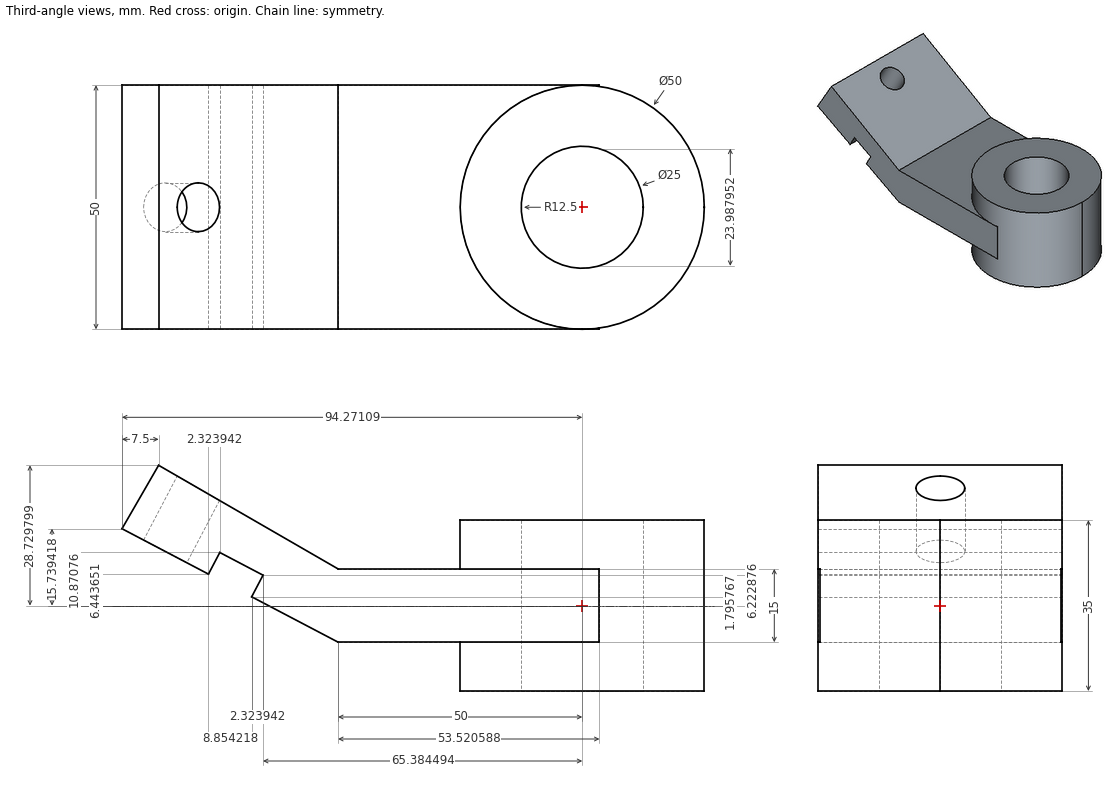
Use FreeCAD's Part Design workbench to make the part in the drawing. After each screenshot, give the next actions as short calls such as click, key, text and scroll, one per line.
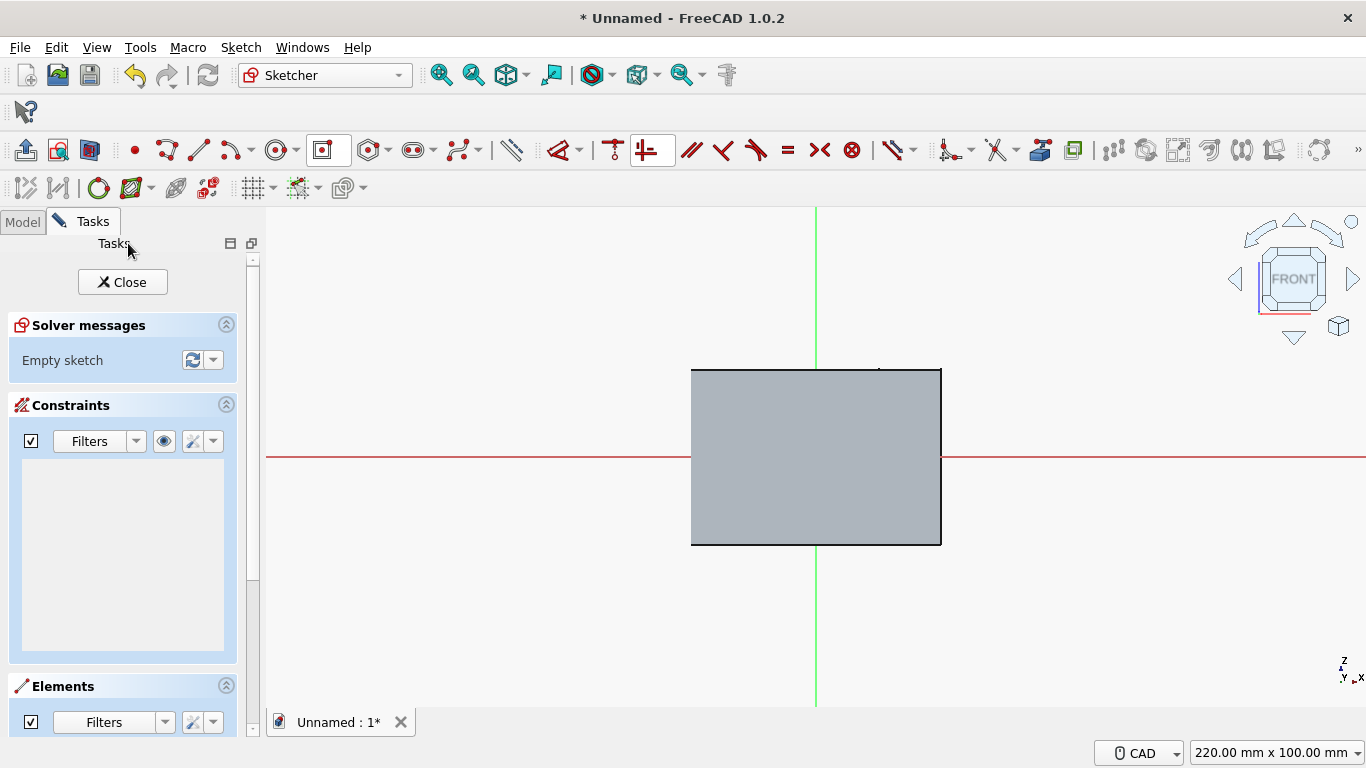
click(90, 150)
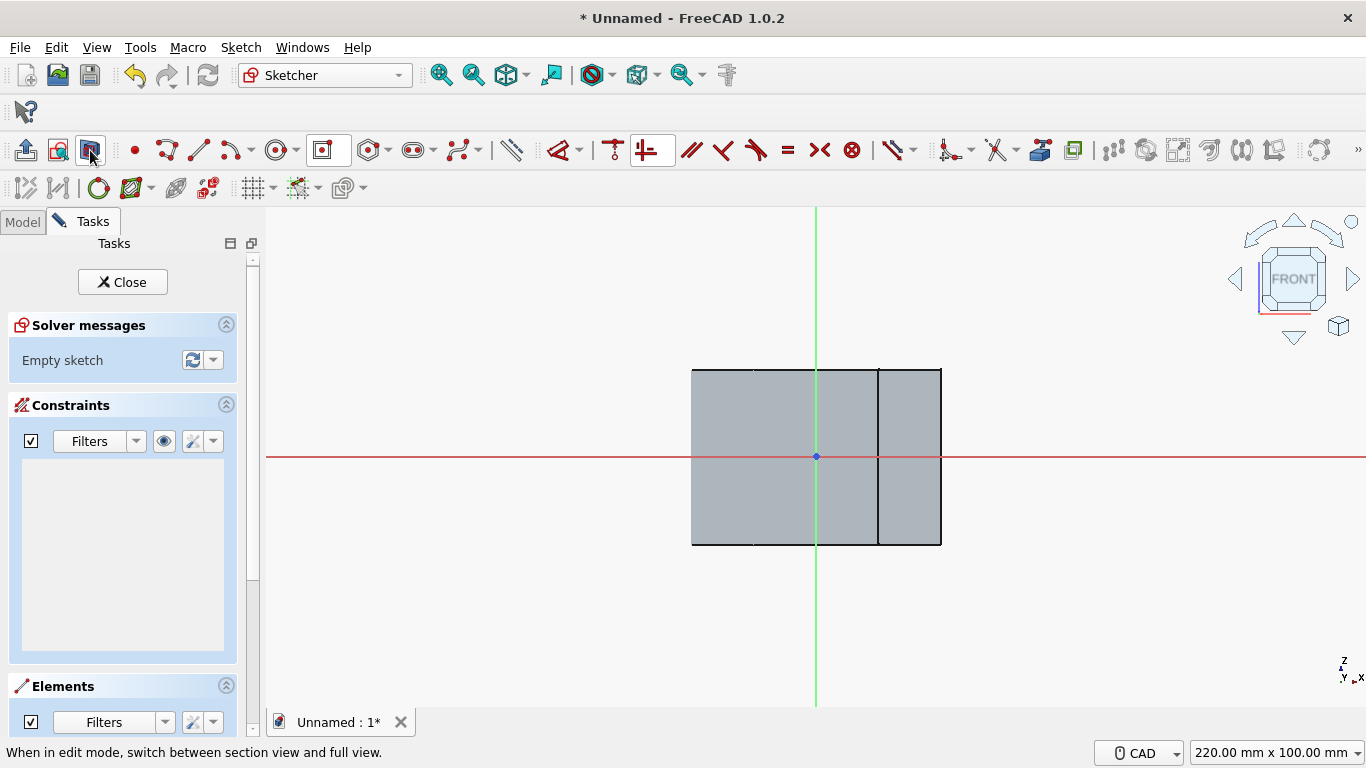
click(168, 150)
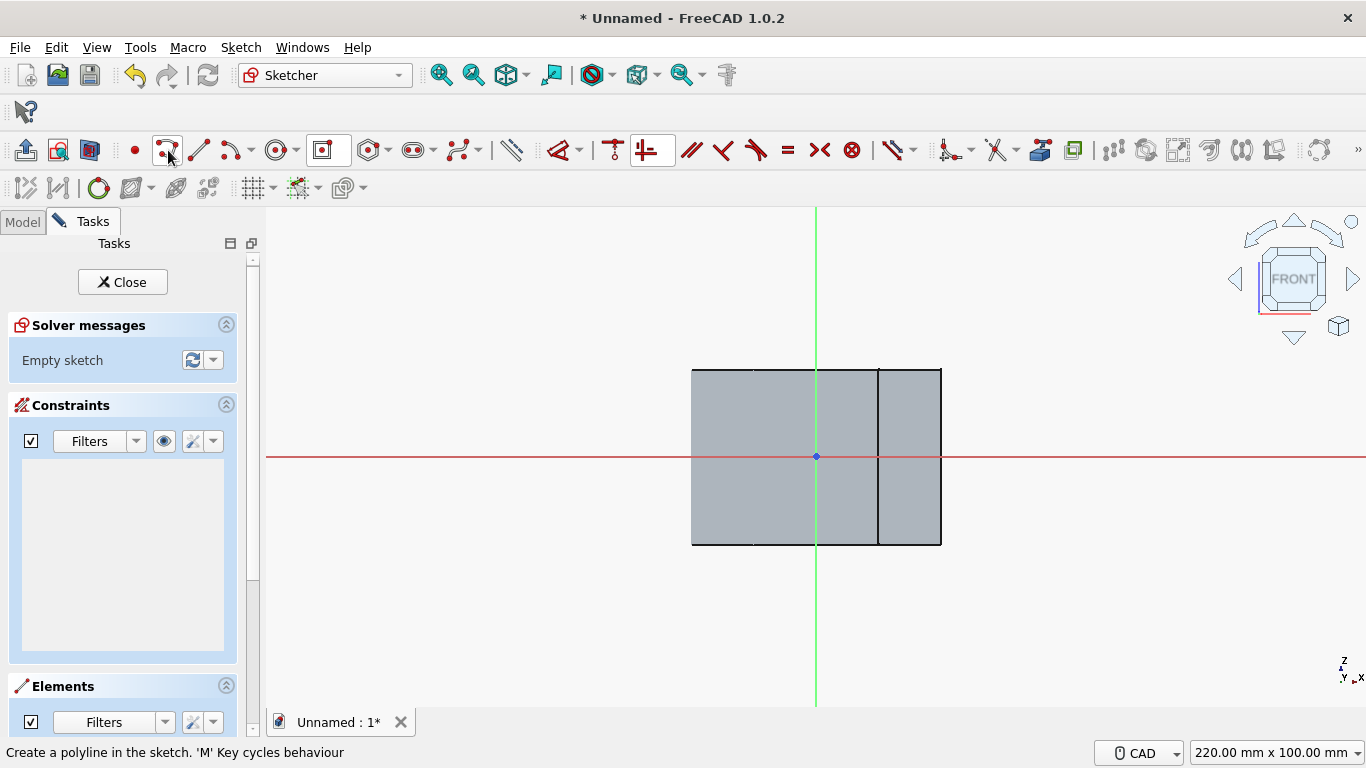
click(834, 494)
click(566, 494)
click(345, 378)
click(382, 313)
click(566, 420)
click(834, 420)
click(834, 495)
key(Escape)
key(Escape)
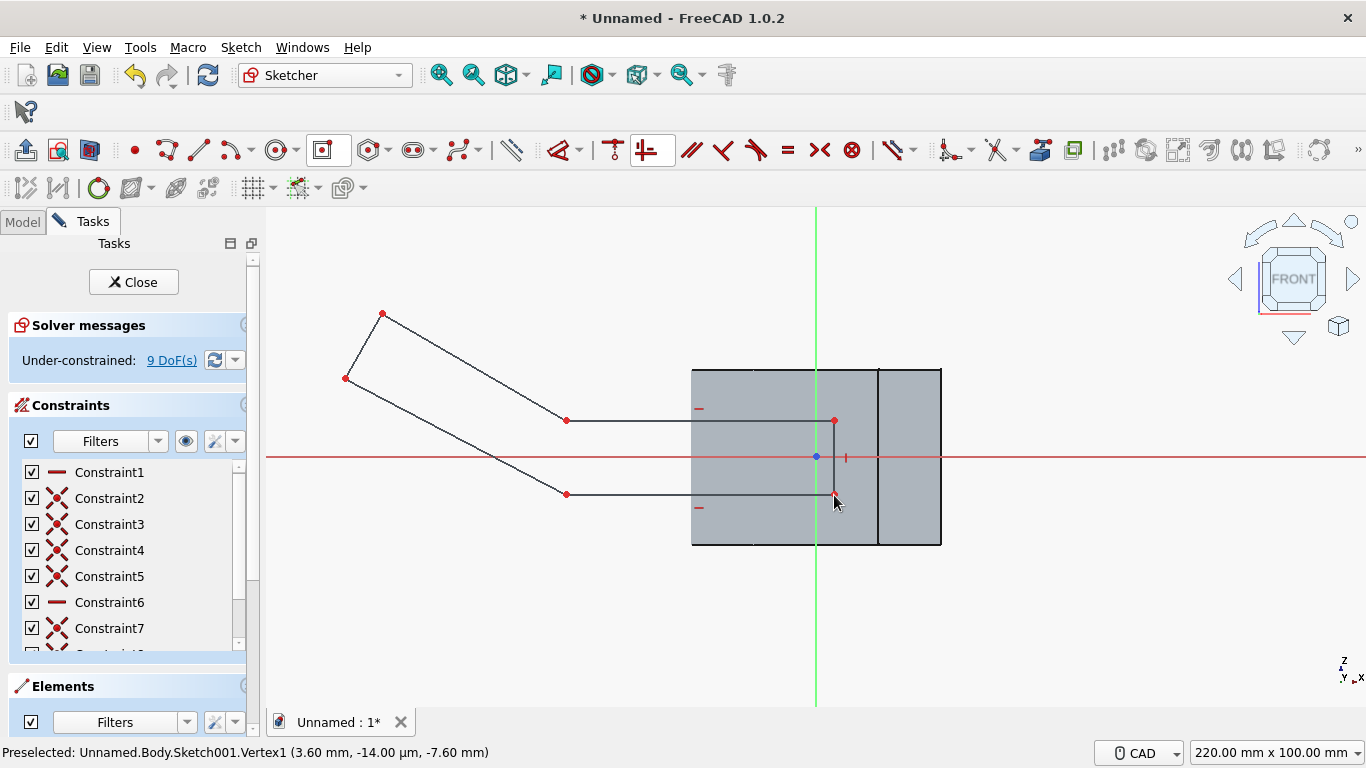
click(566, 495)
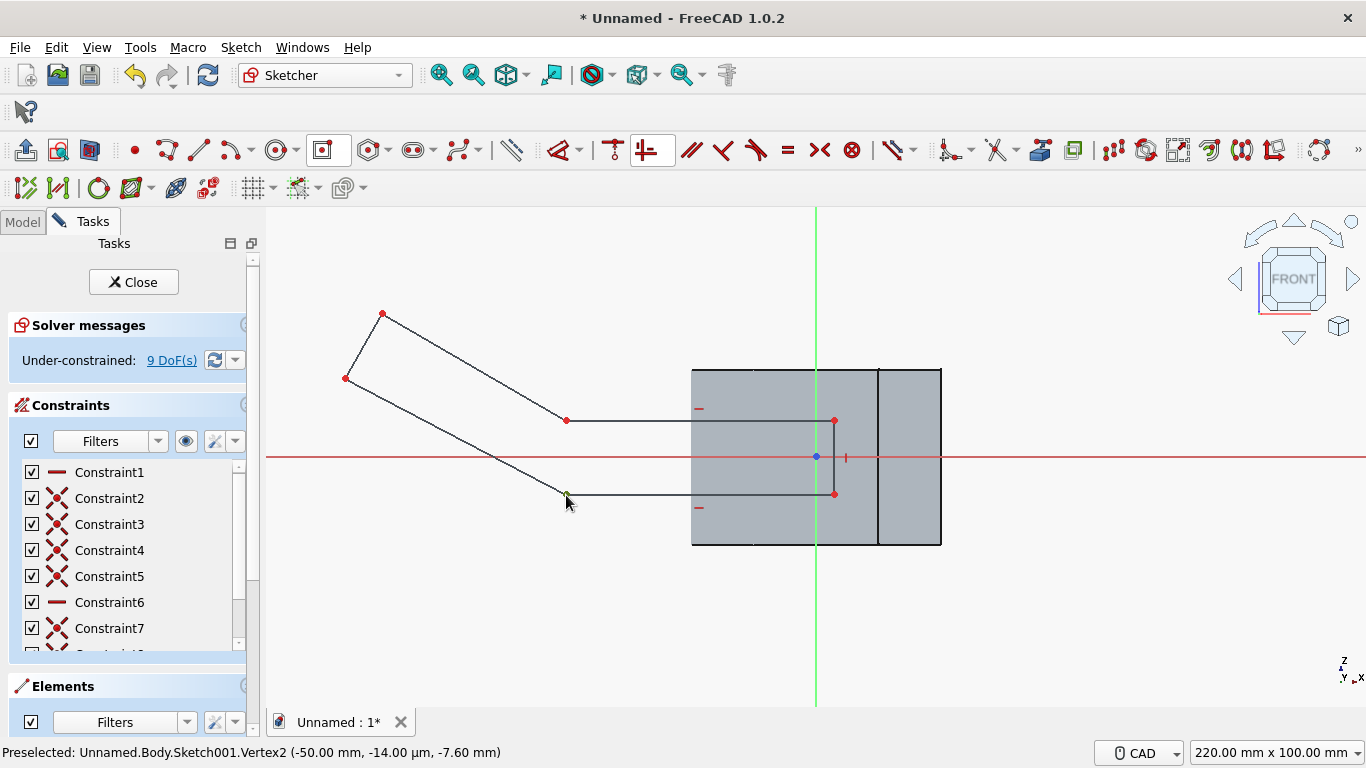
click(566, 421)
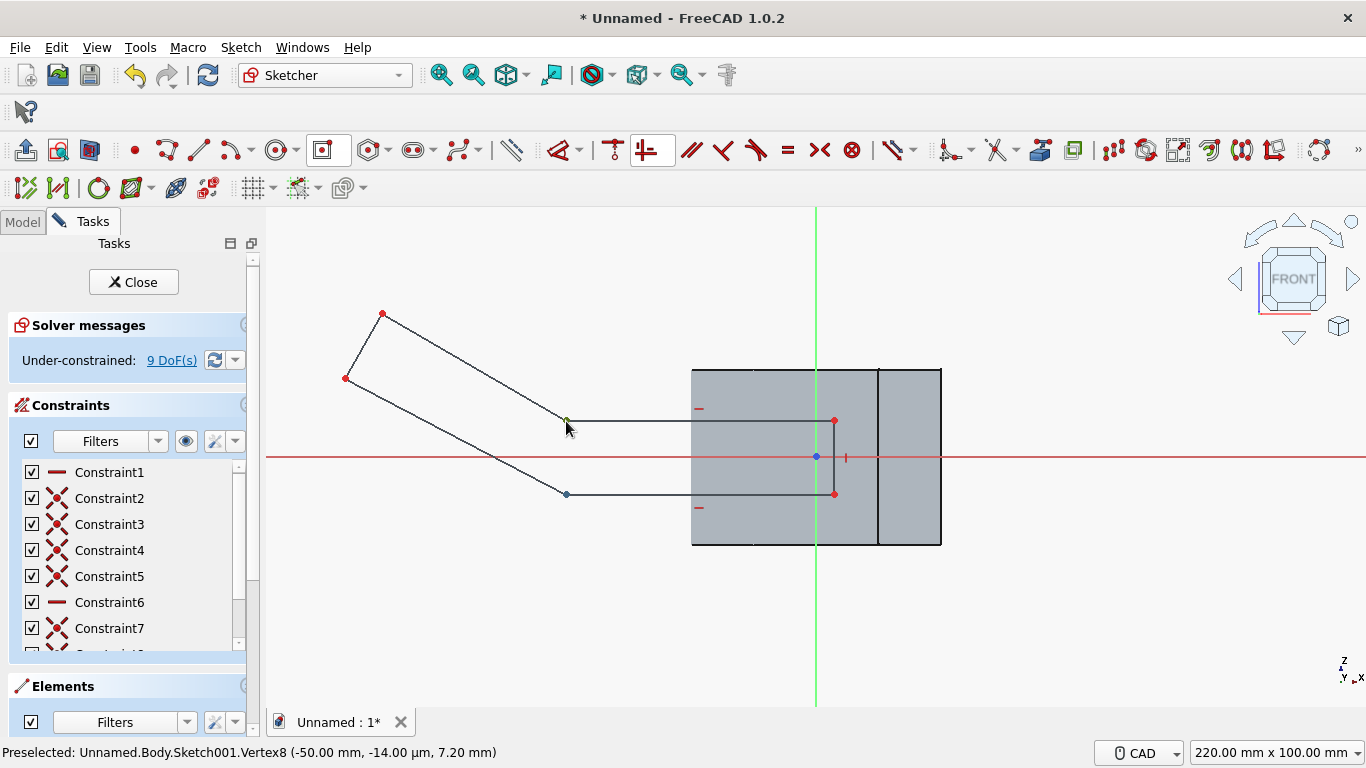
click(359, 457)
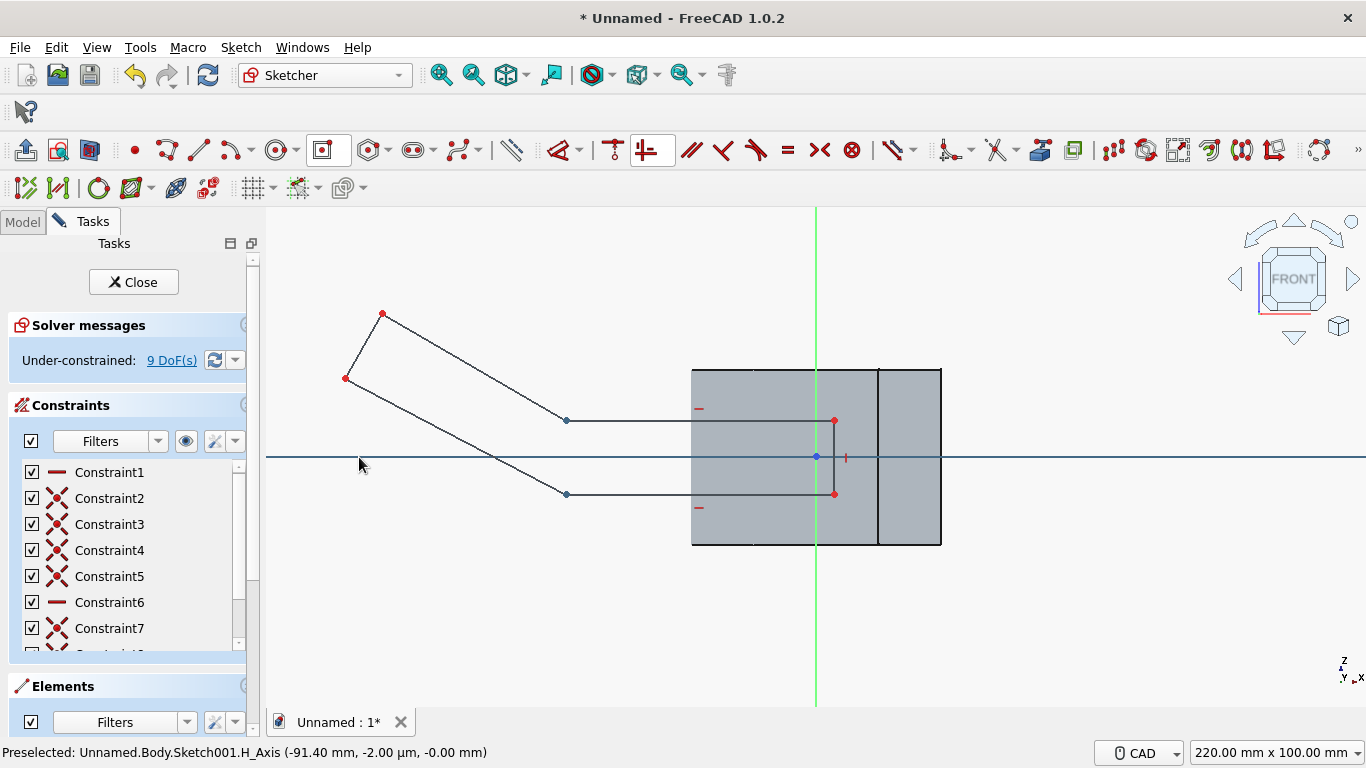
click(820, 150)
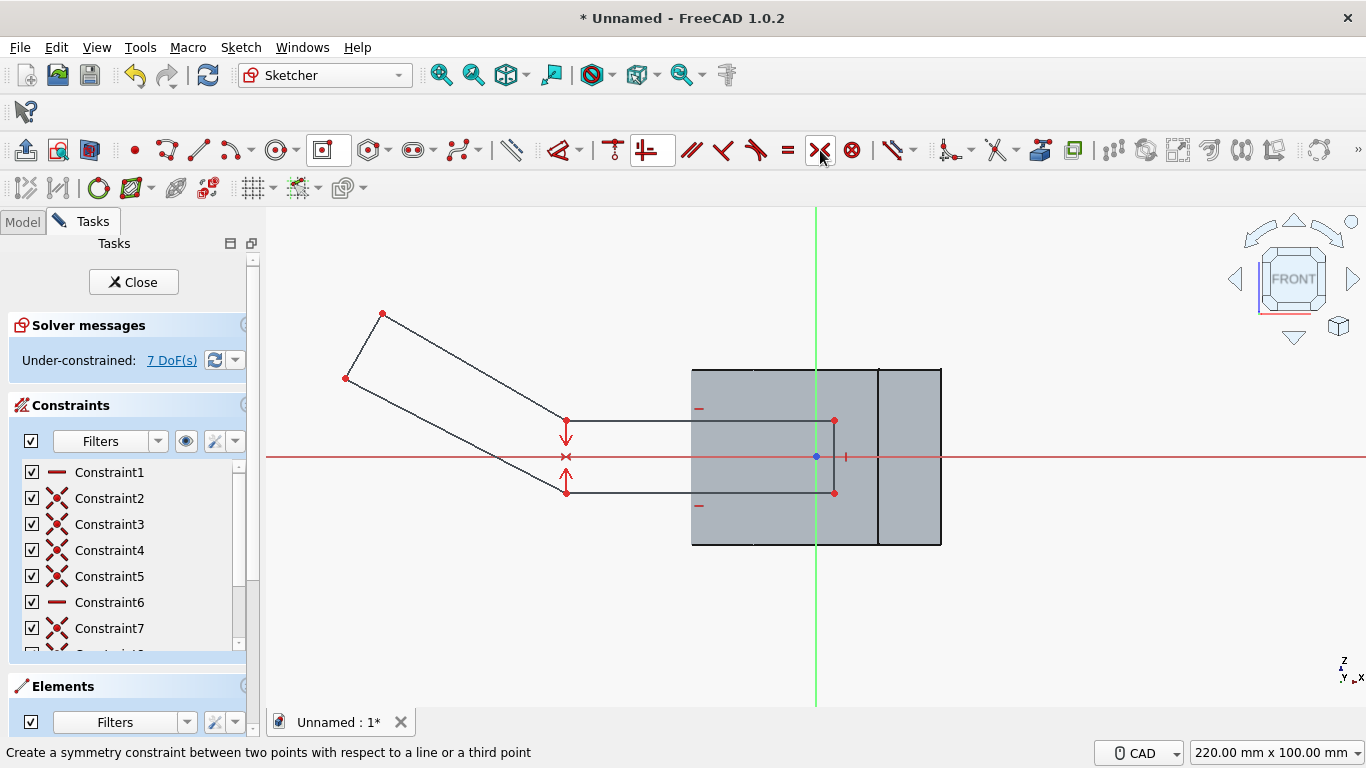
click(558, 150)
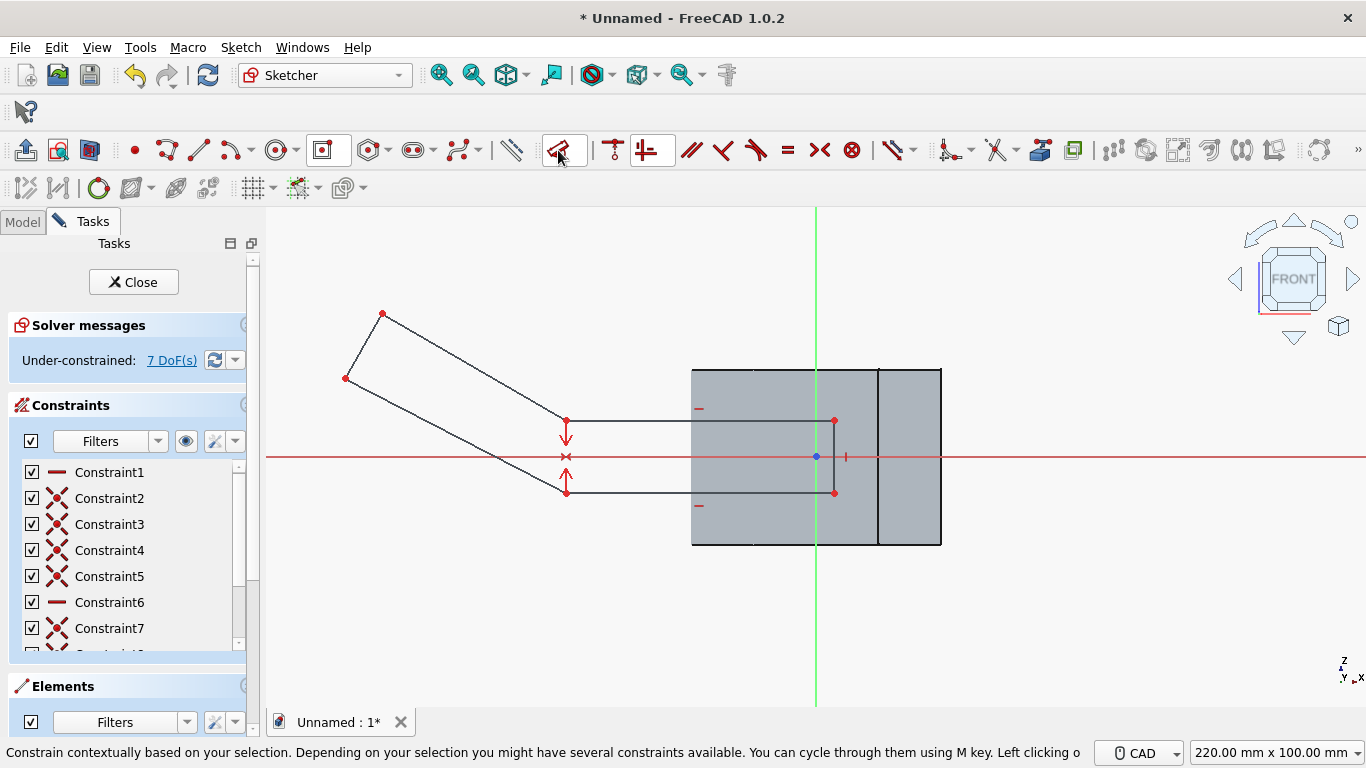
click(834, 442)
click(868, 440)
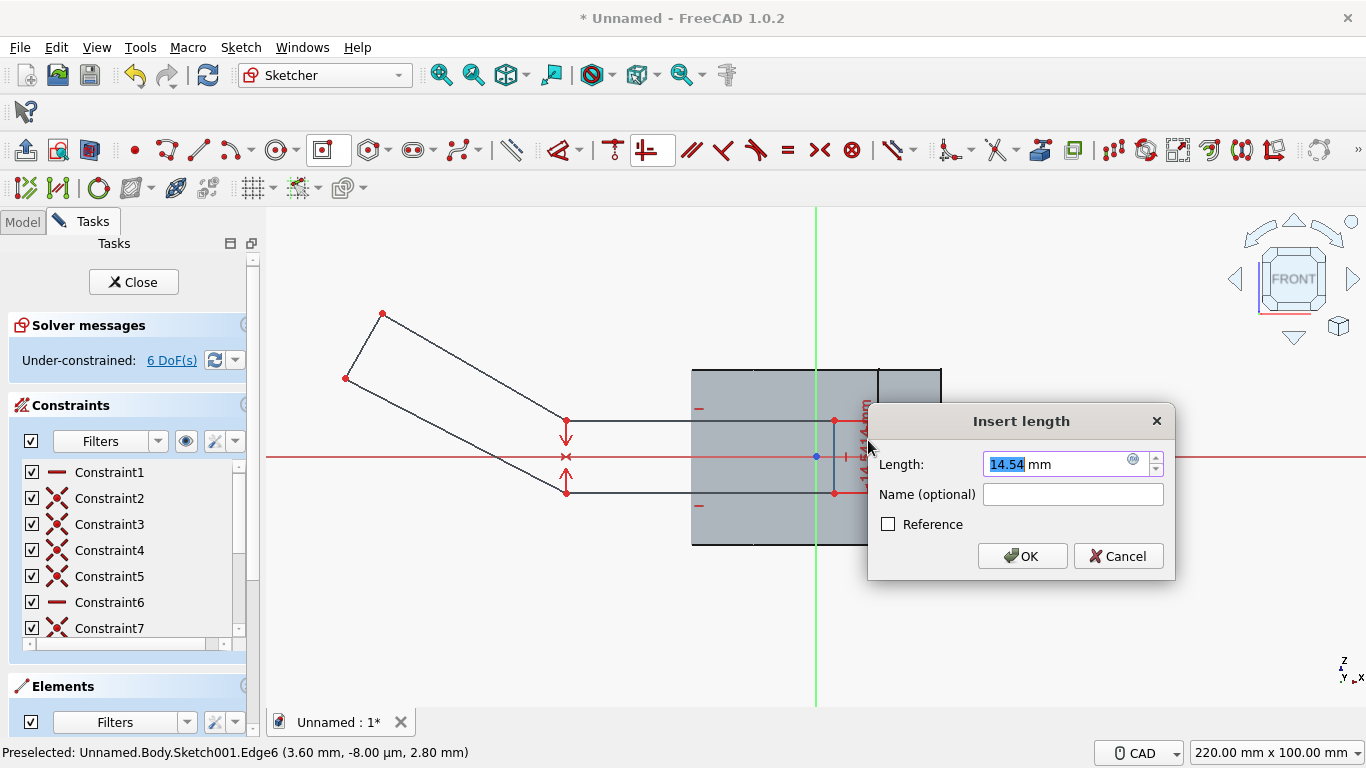
text(15)
key(Return)